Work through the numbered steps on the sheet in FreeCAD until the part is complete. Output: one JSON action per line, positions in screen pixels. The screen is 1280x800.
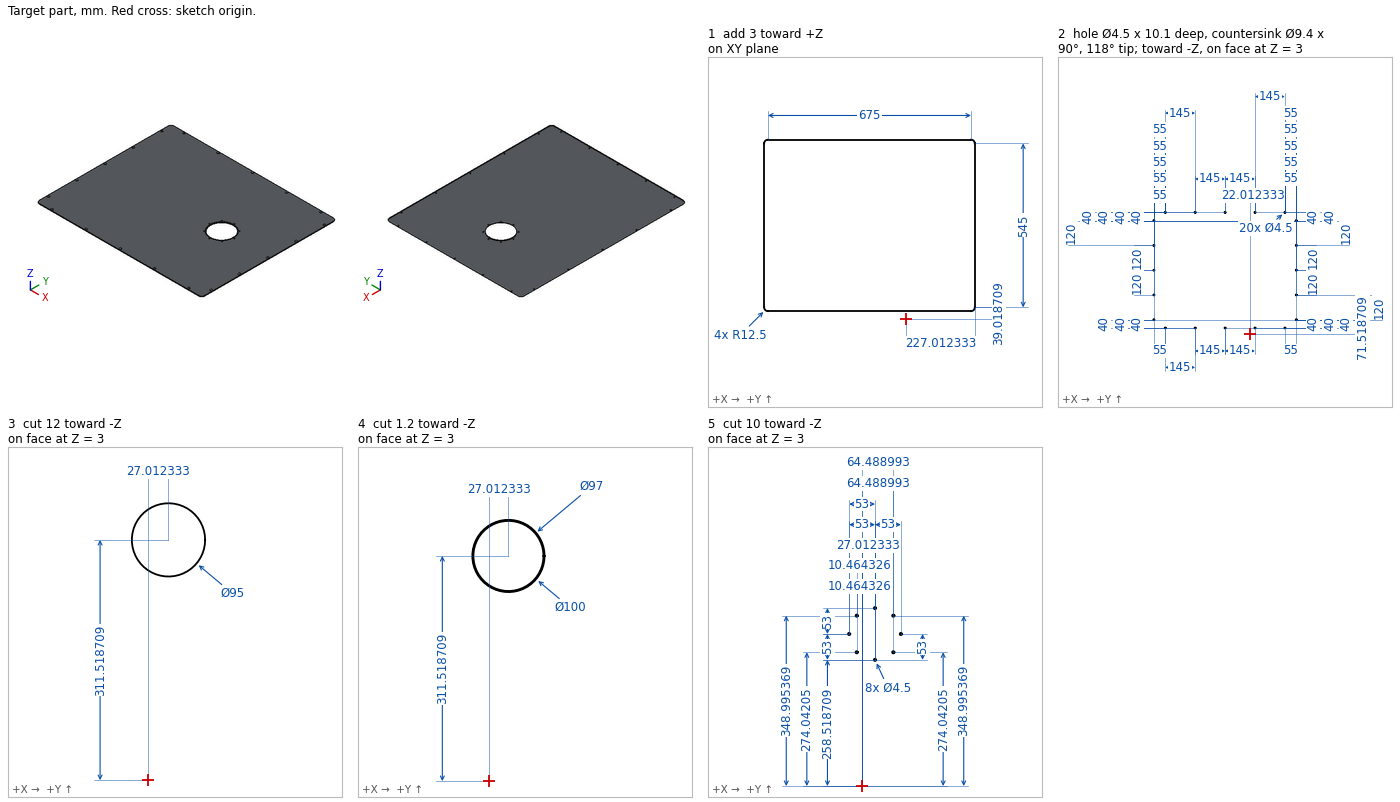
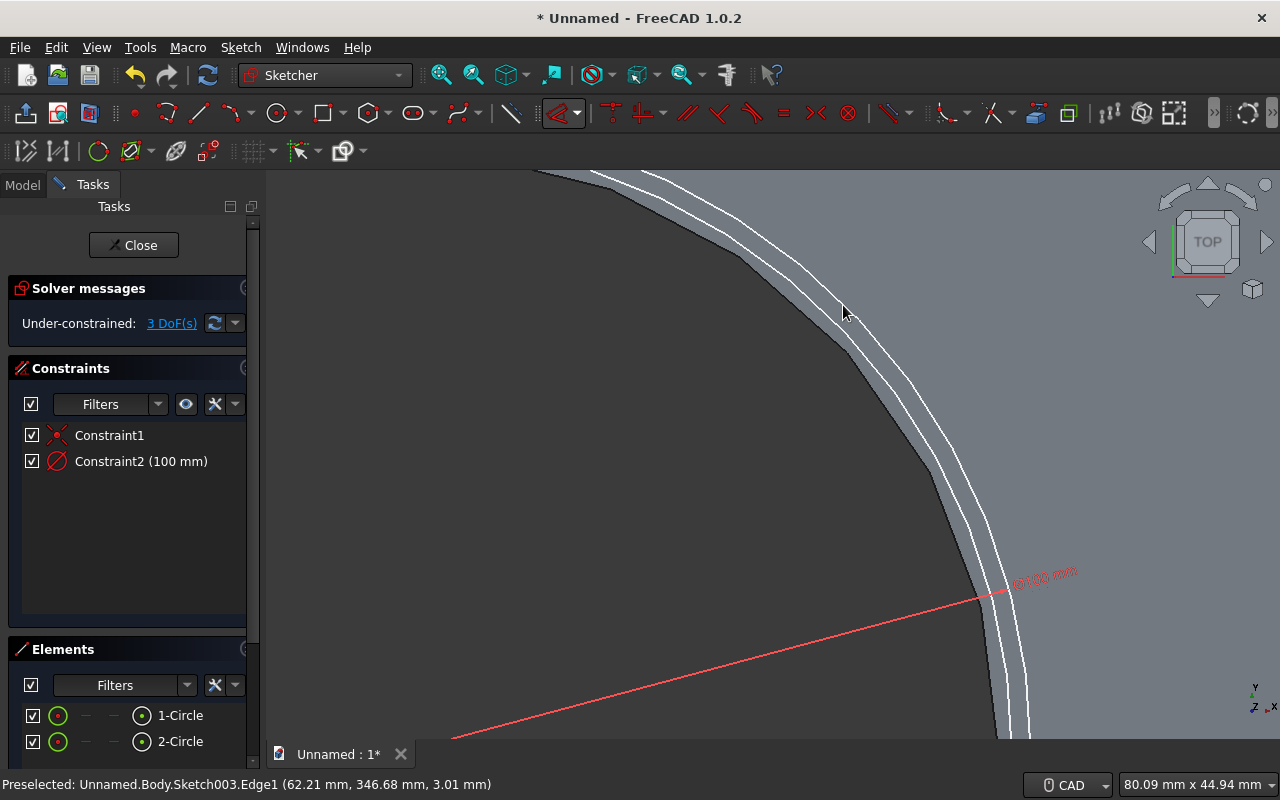
{"action": "left_click", "coordinate": [831, 318]}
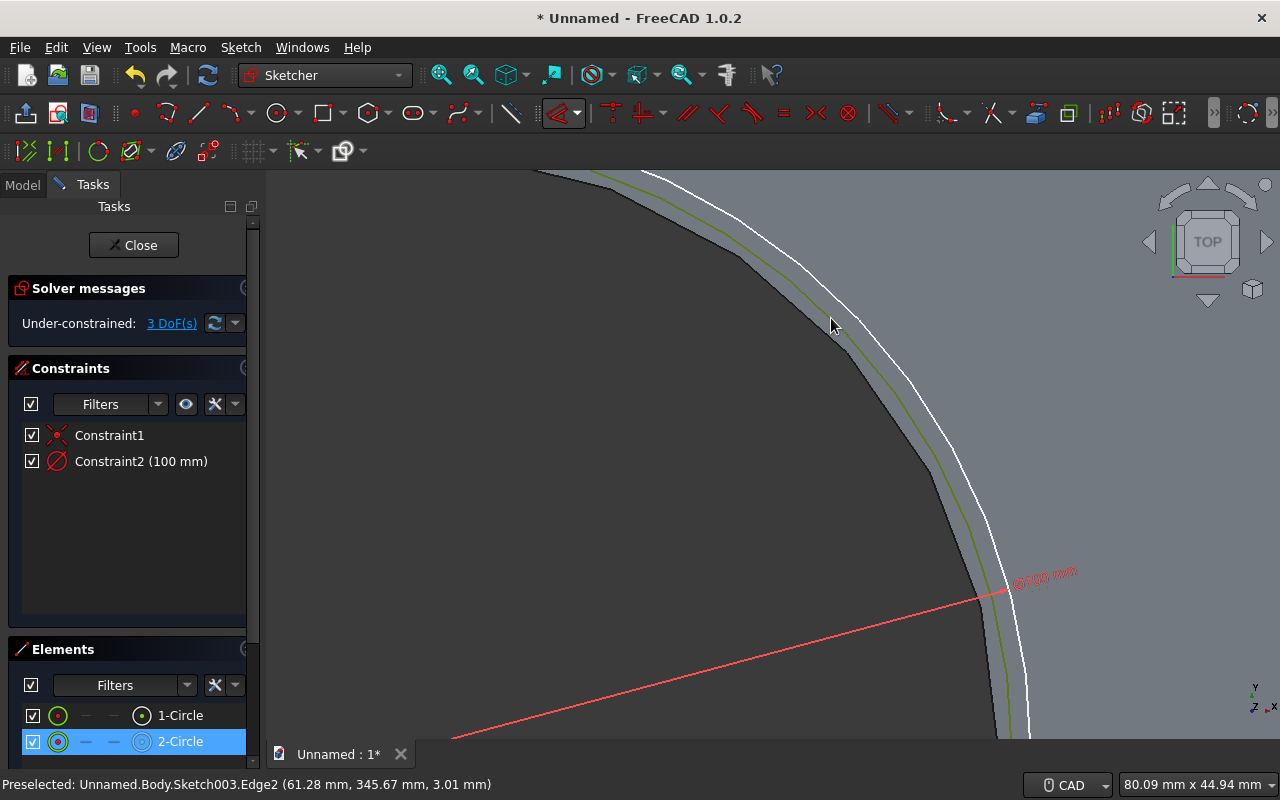
{"action": "left_click", "coordinate": [580, 114]}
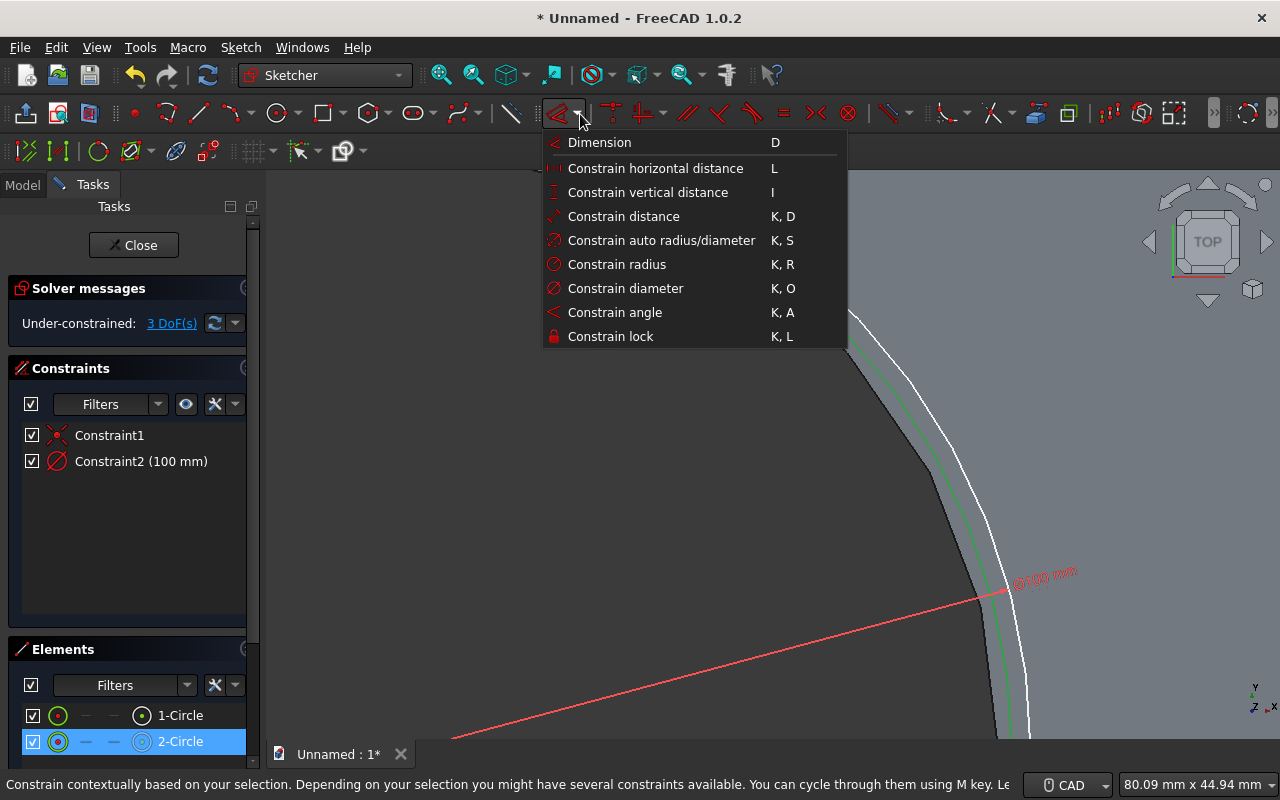
{"action": "left_click", "coordinate": [695, 288]}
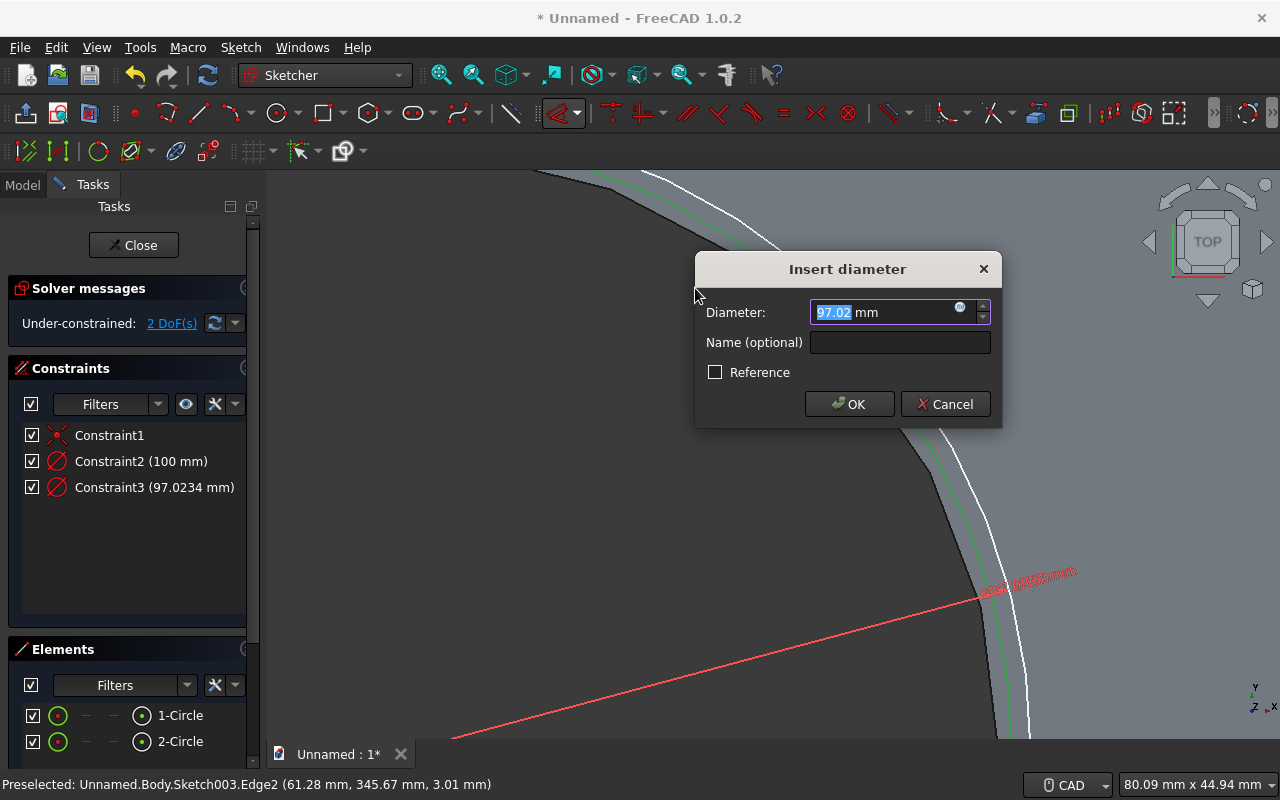
{"action": "type", "text": "97"}
{"action": "key", "text": "Return"}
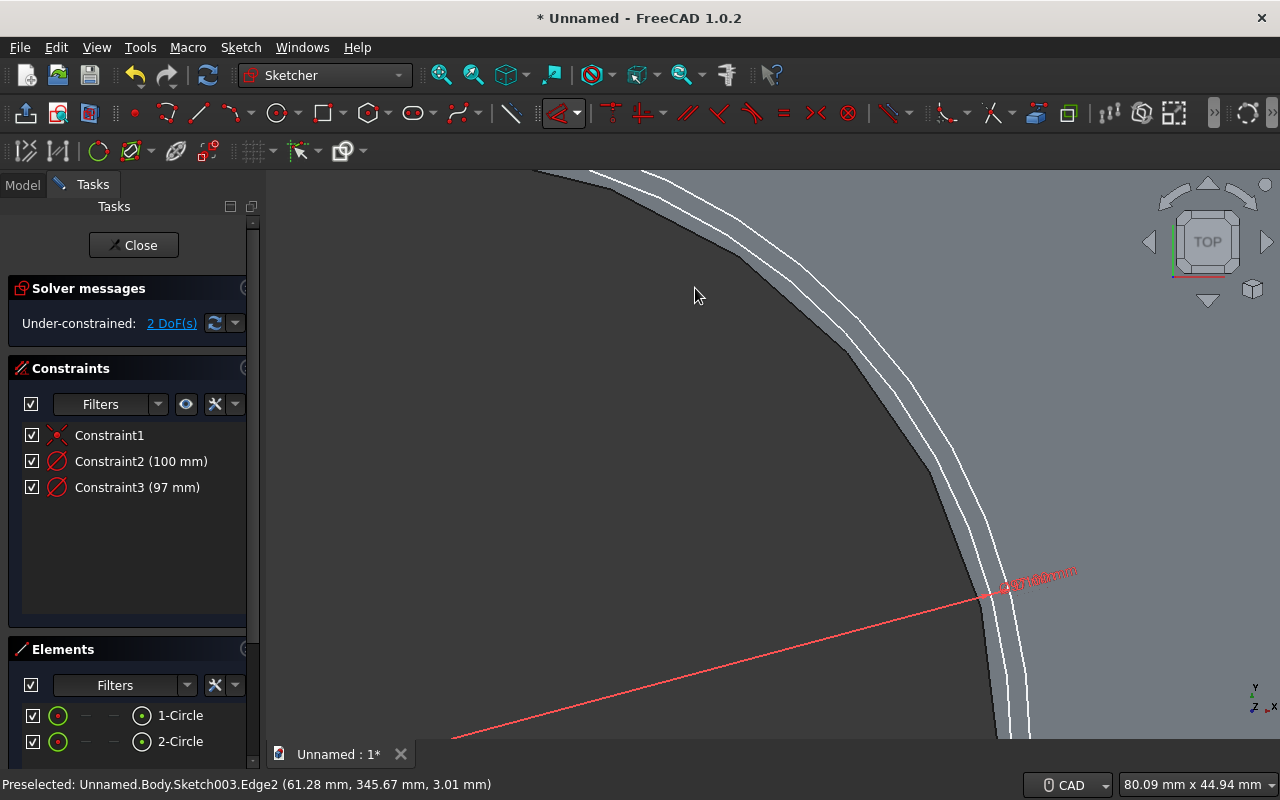
{"action": "scroll", "coordinate": [837, 326], "scroll_direction": "down", "scroll_amount": 6}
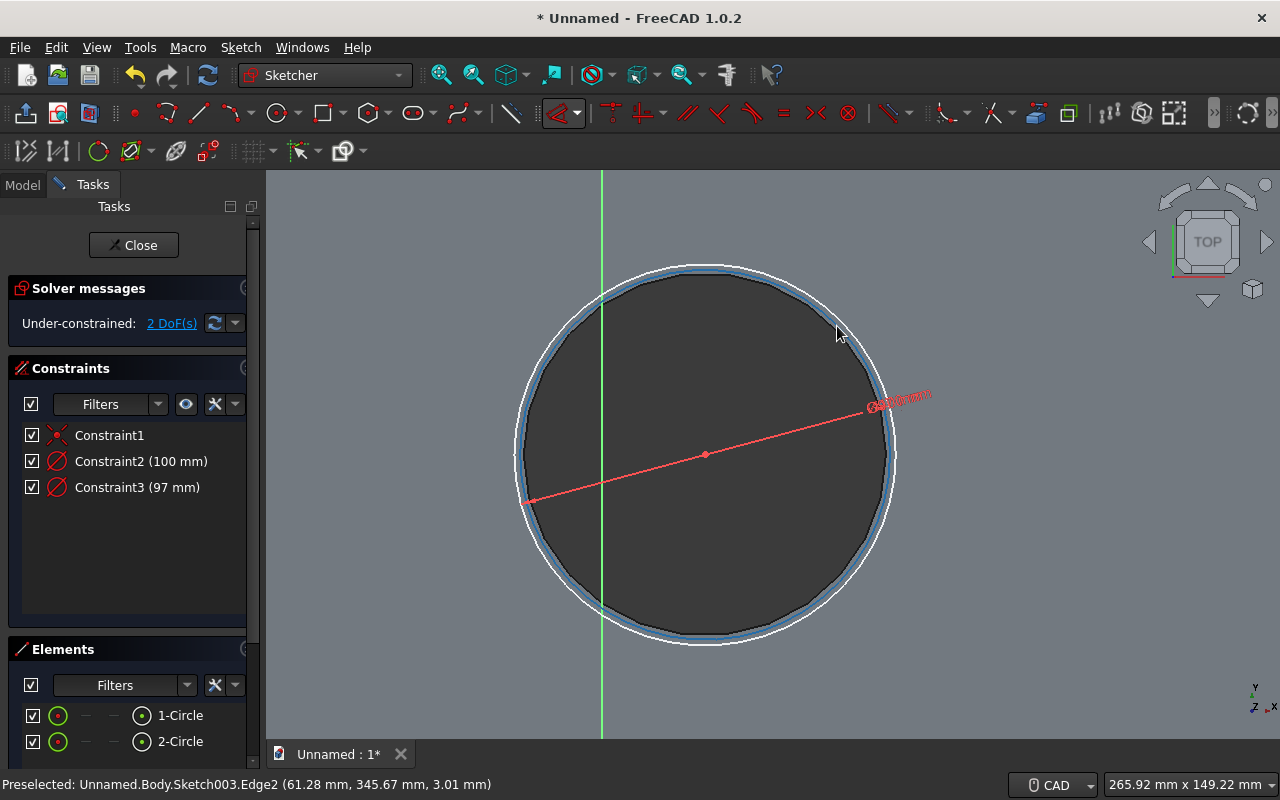
{"action": "left_click", "coordinate": [705, 455]}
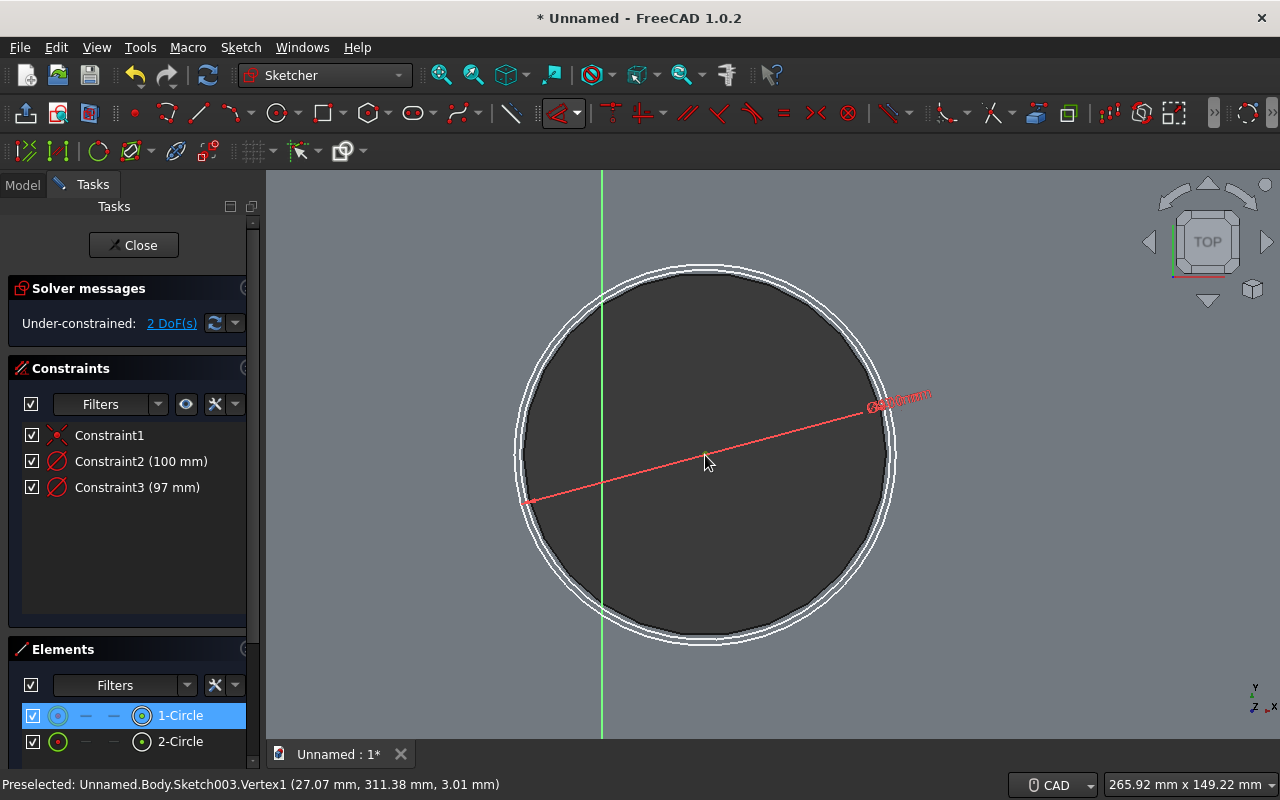
{"action": "left_click", "coordinate": [580, 114]}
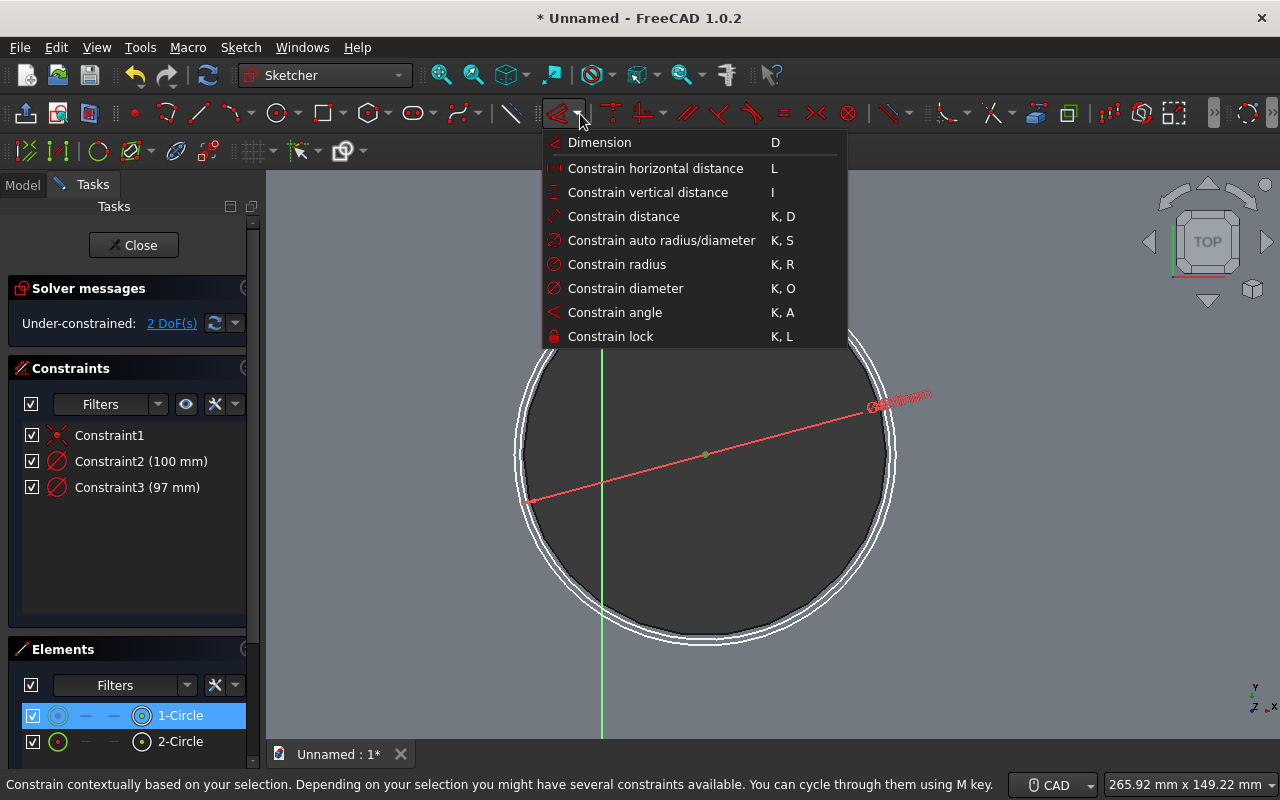
{"action": "left_click", "coordinate": [695, 168]}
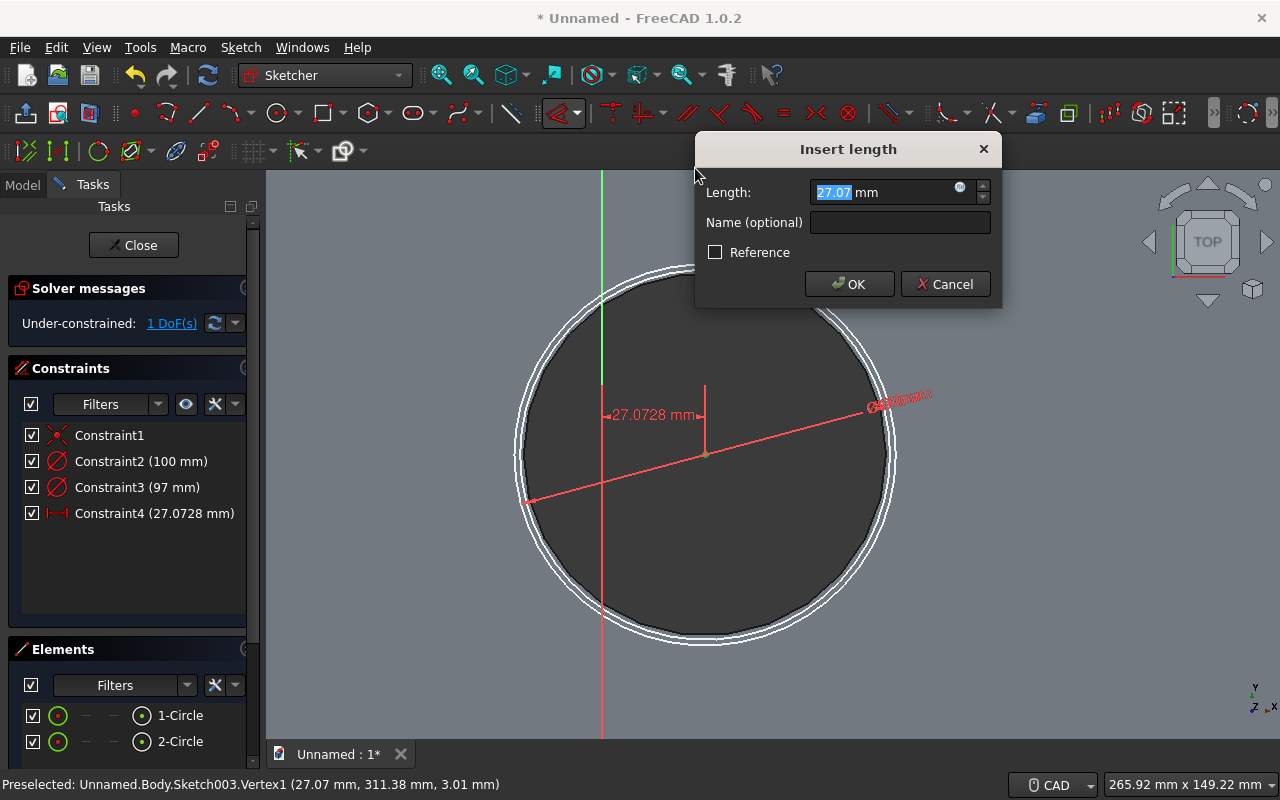
{"action": "type", "text": "27.012333"}
{"action": "key", "text": "Return"}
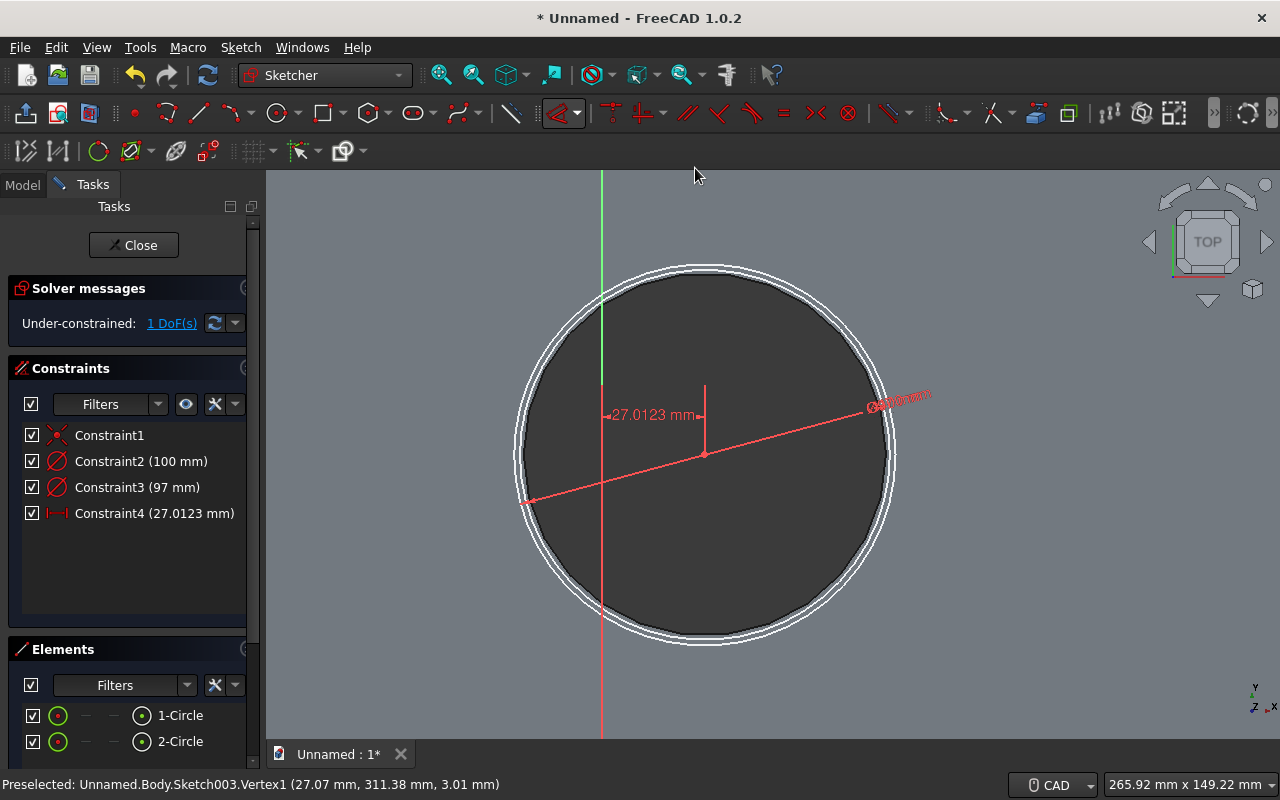
{"action": "left_click", "coordinate": [705, 455]}